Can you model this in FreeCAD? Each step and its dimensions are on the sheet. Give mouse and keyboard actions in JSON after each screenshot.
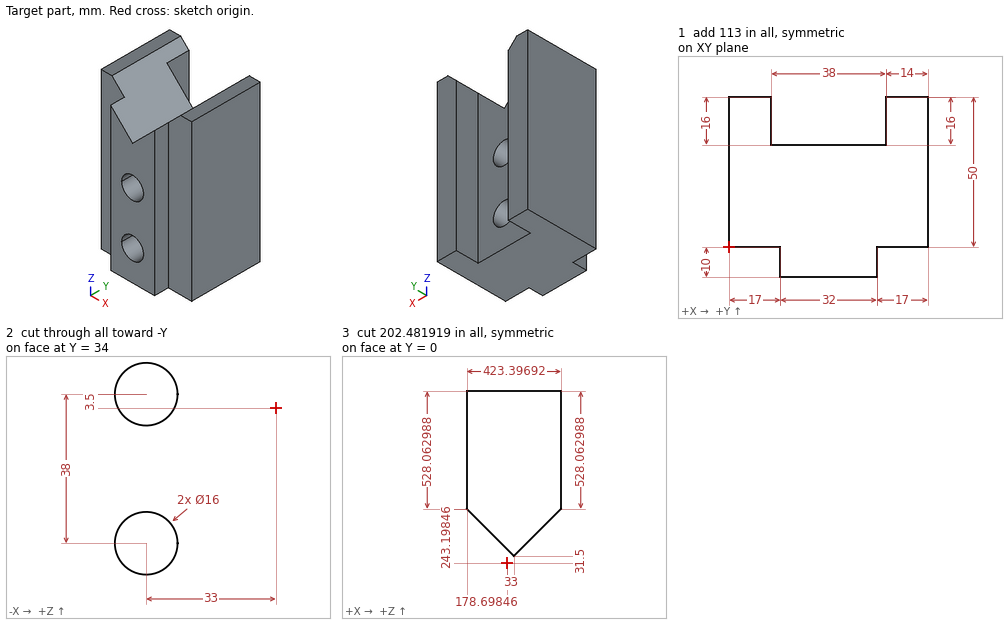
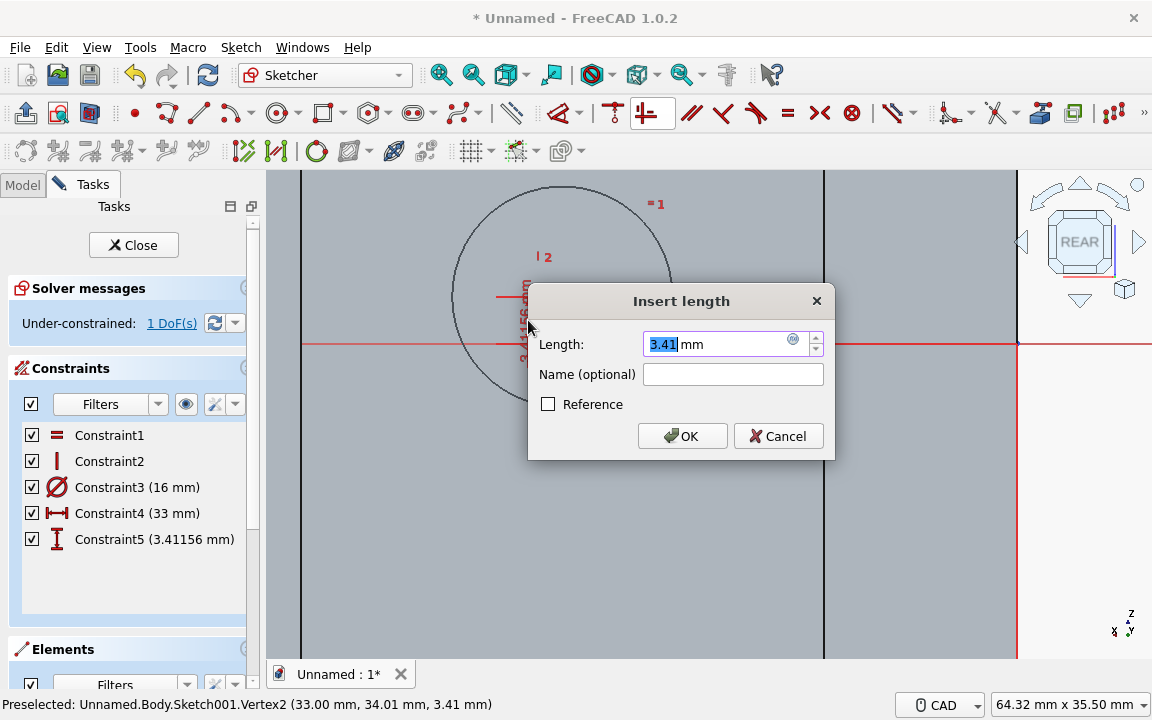
{"action": "type", "text": "3.5"}
{"action": "key", "text": "Return"}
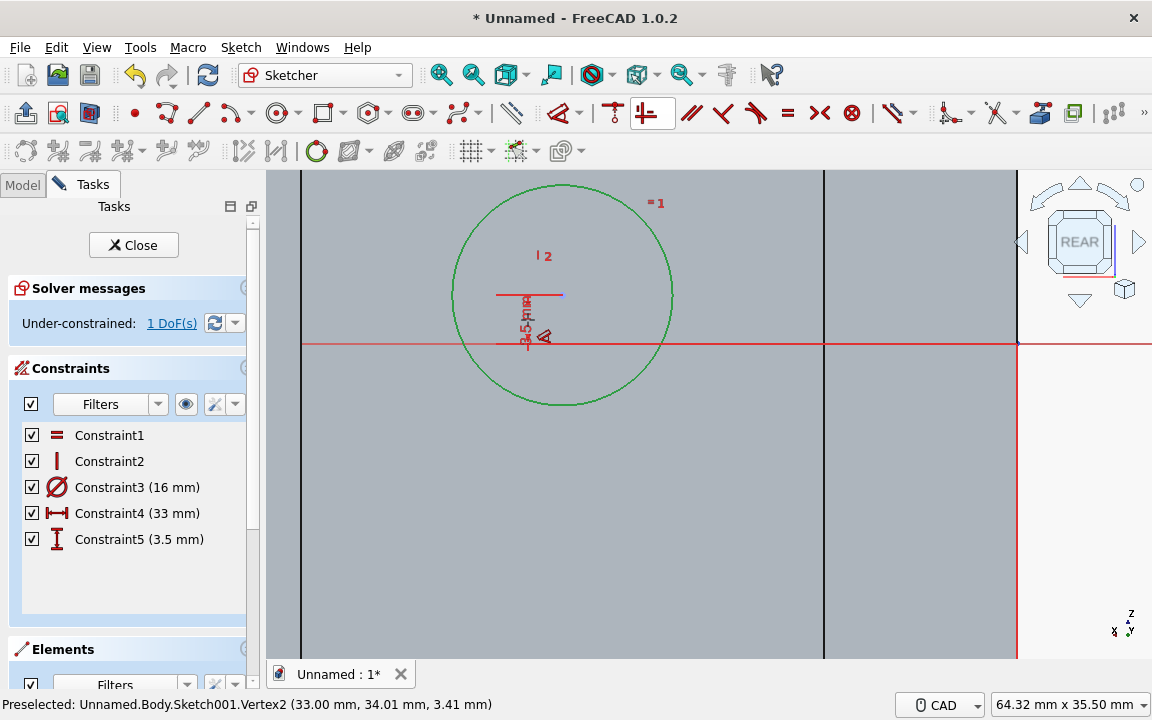
{"action": "scroll", "coordinate": [564, 298], "scroll_direction": "down", "scroll_amount": 4}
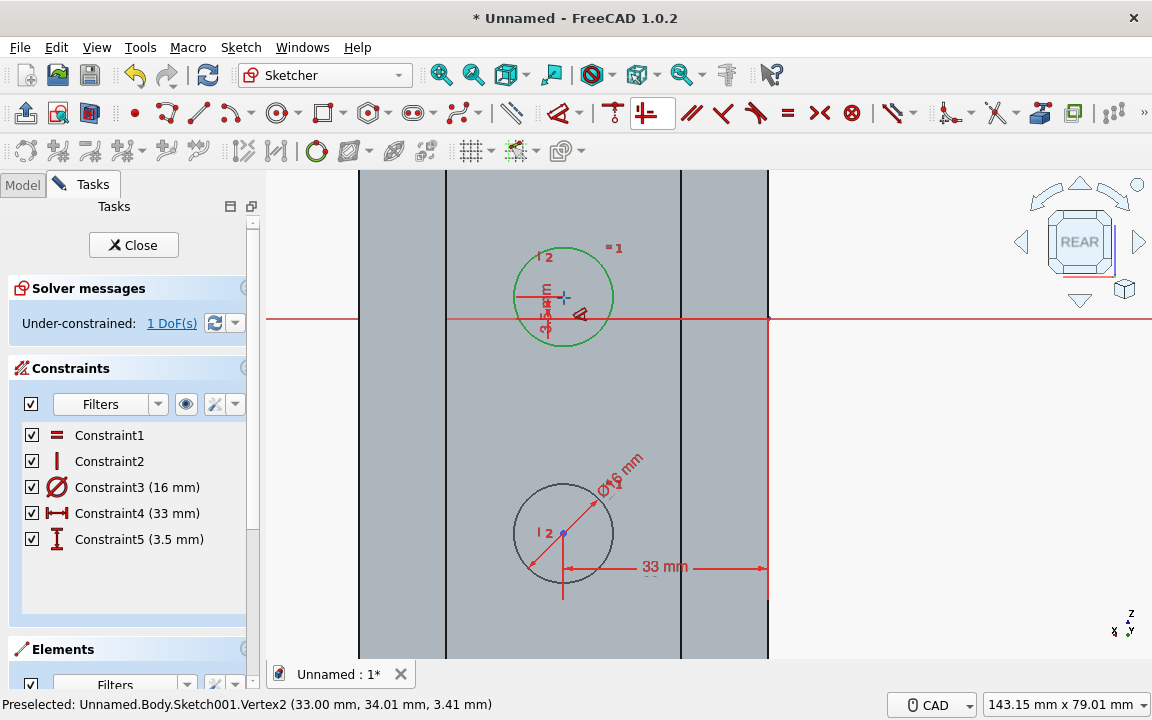
{"action": "left_click", "coordinate": [563, 534]}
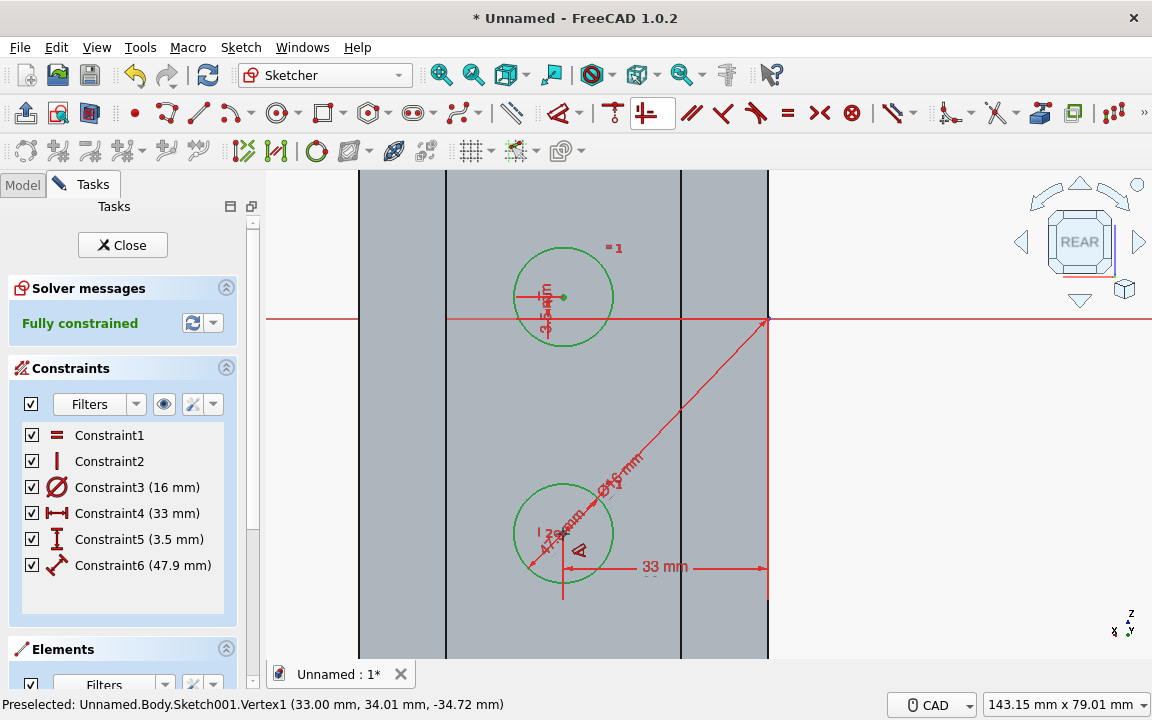
{"action": "left_click", "coordinate": [563, 297]}
{"action": "left_click", "coordinate": [529, 415]}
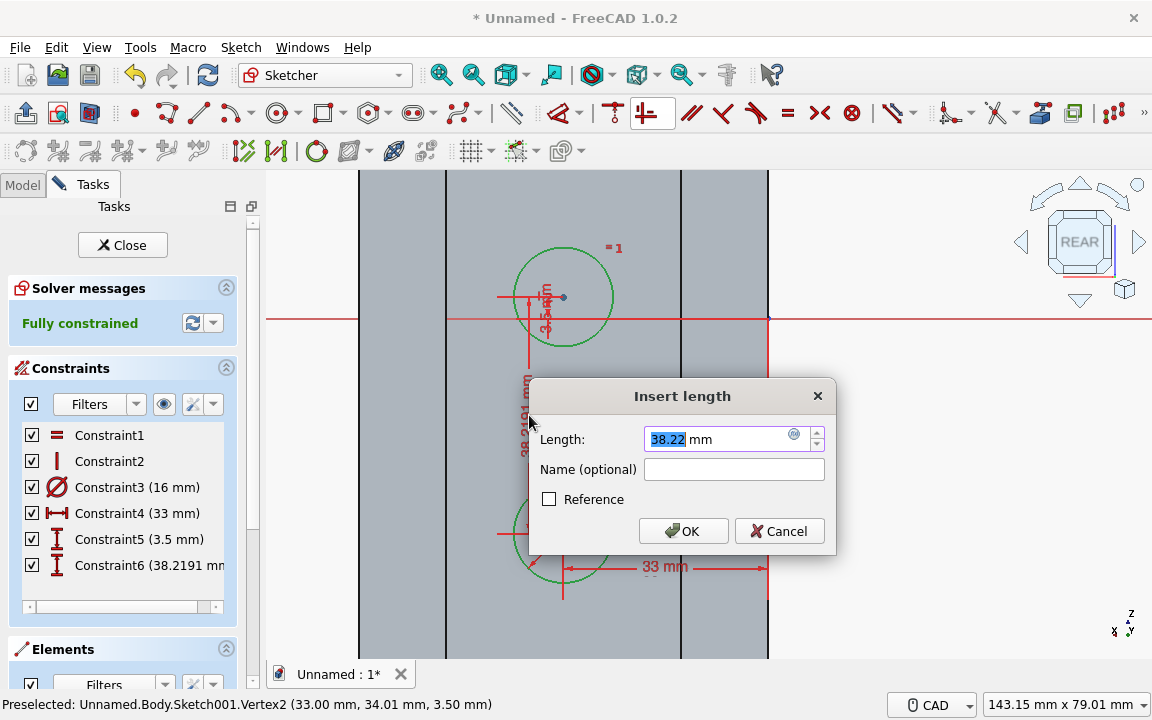
{"action": "type", "text": "38"}
{"action": "key", "text": "Return"}
{"action": "key", "text": "Escape"}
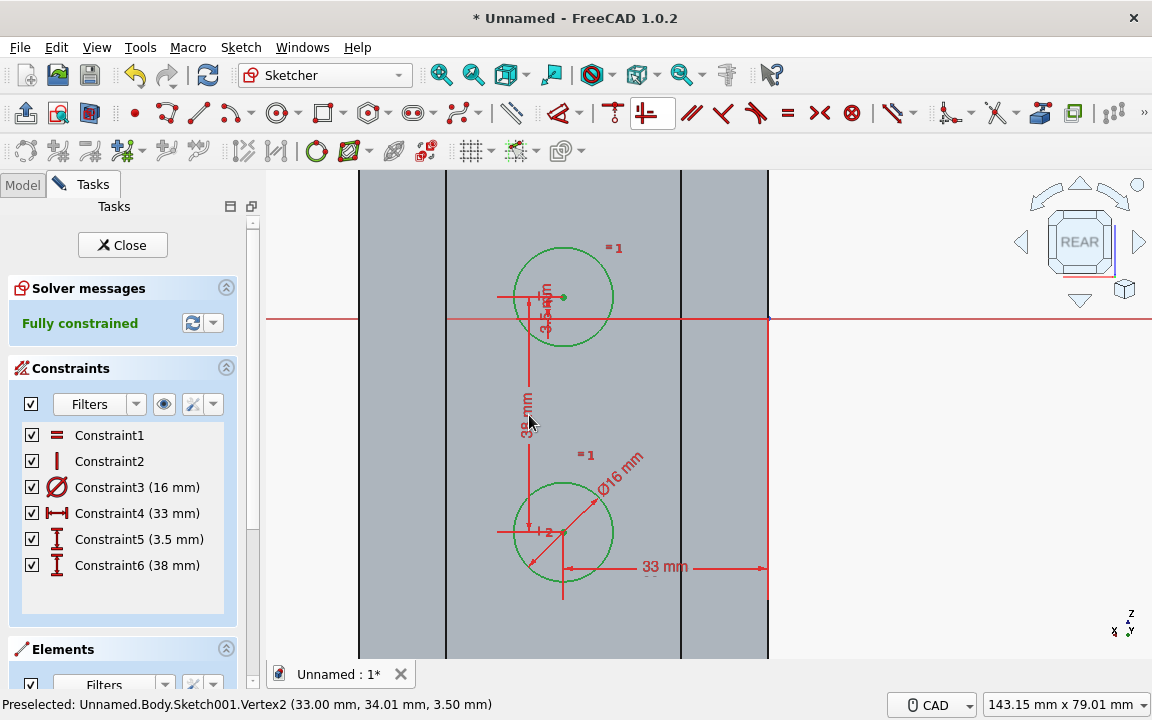
{"action": "left_click", "coordinate": [123, 245]}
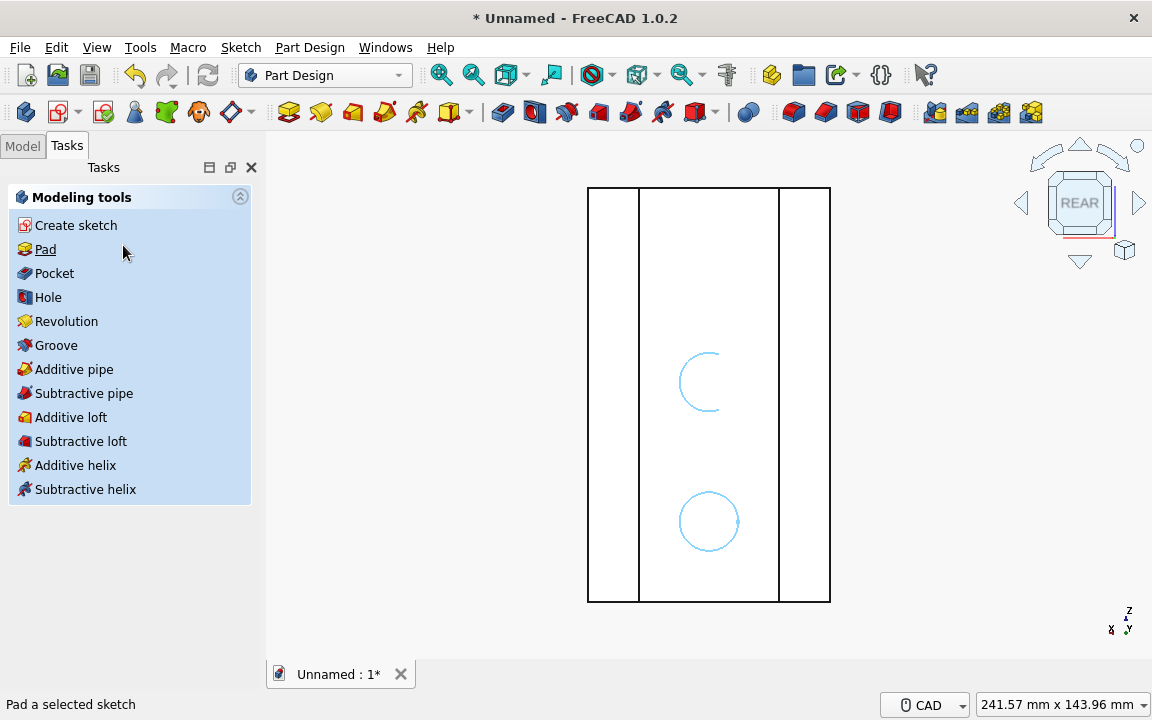
{"action": "left_click", "coordinate": [504, 112]}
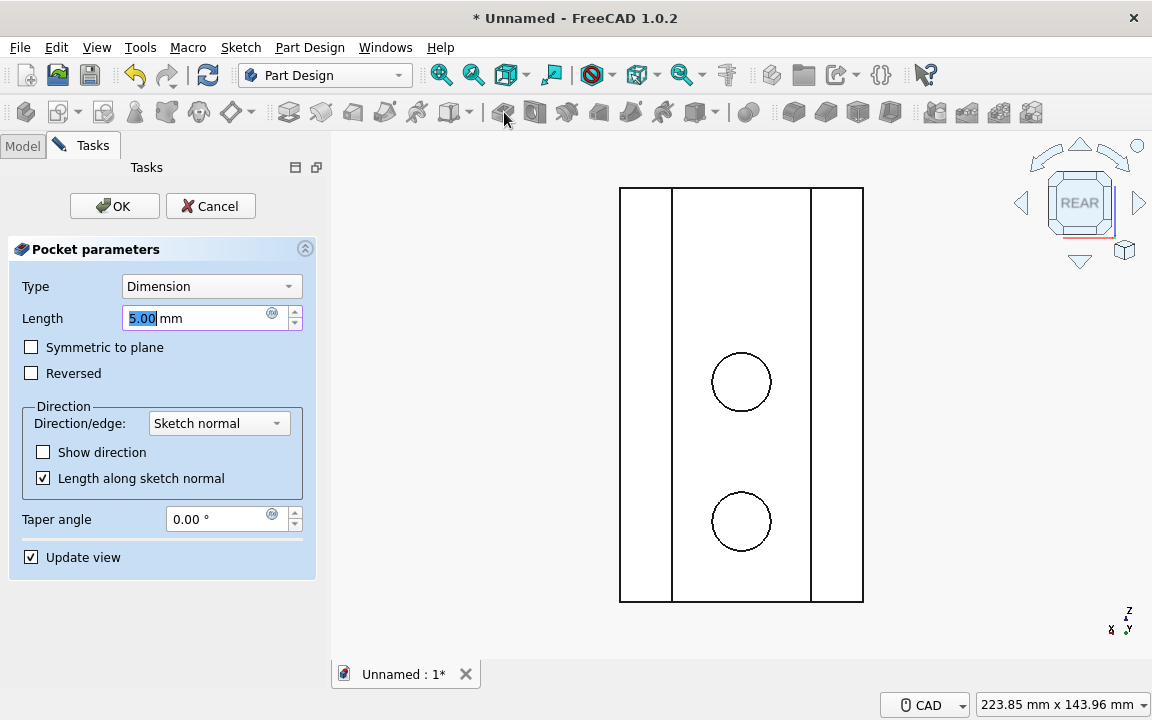
{"action": "left_click", "coordinate": [212, 286]}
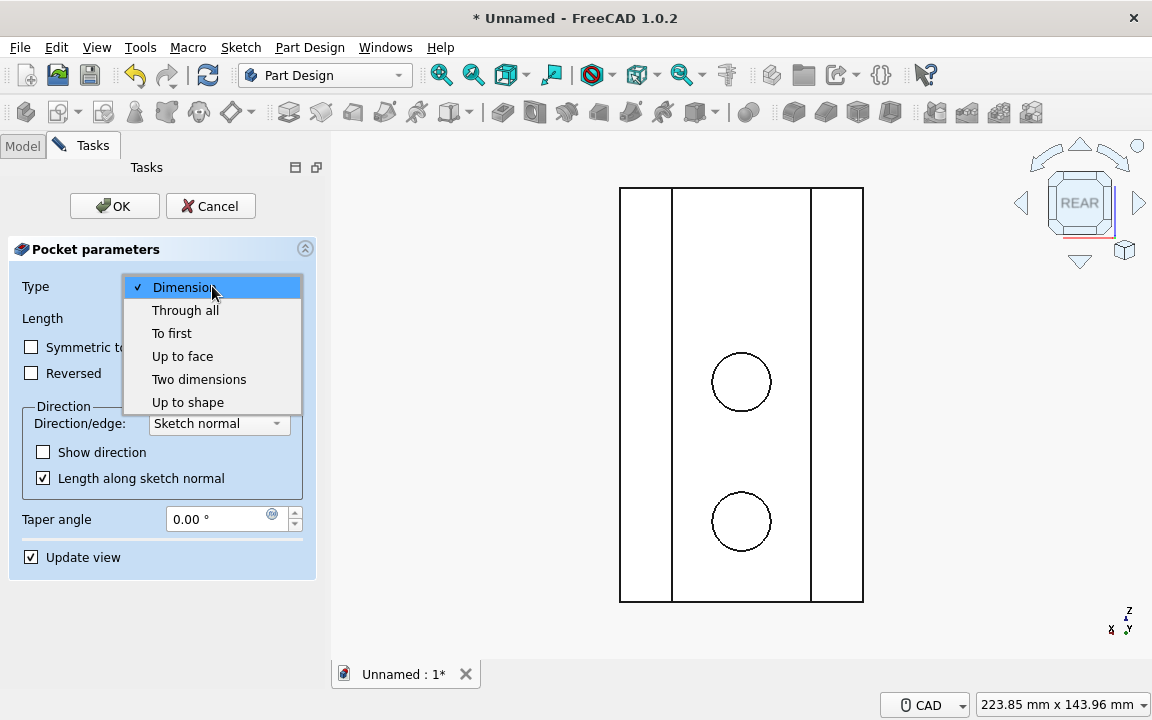
{"action": "left_click", "coordinate": [212, 310]}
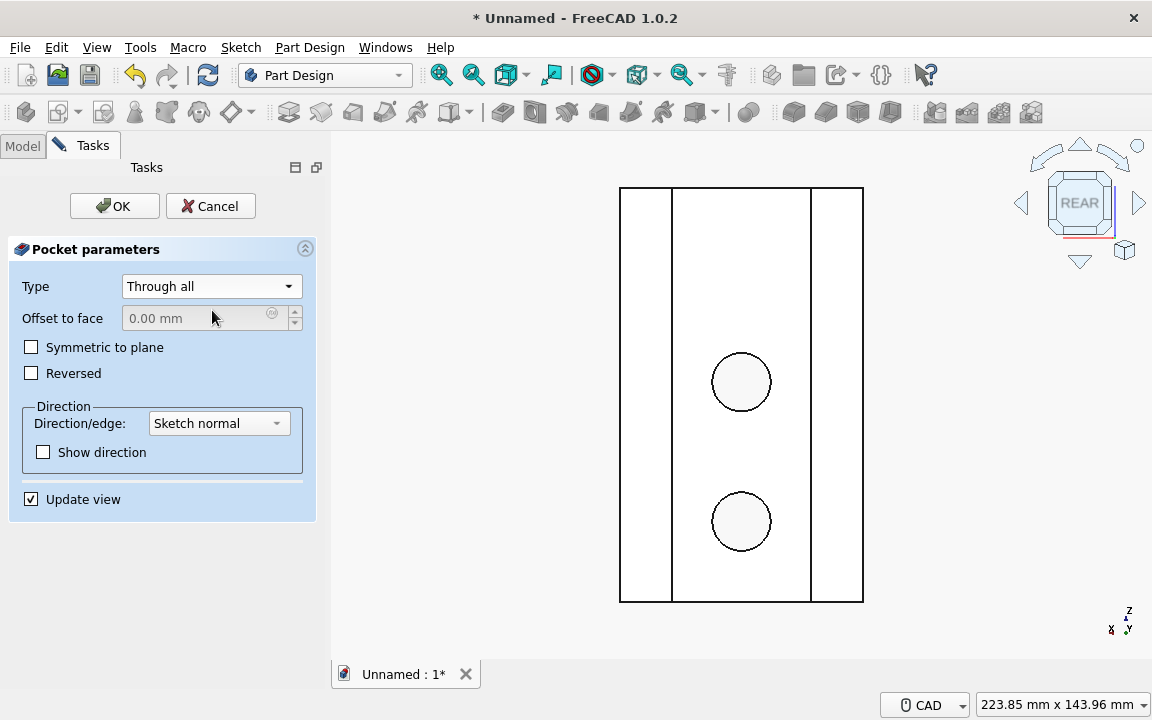
{"action": "left_click", "coordinate": [115, 206]}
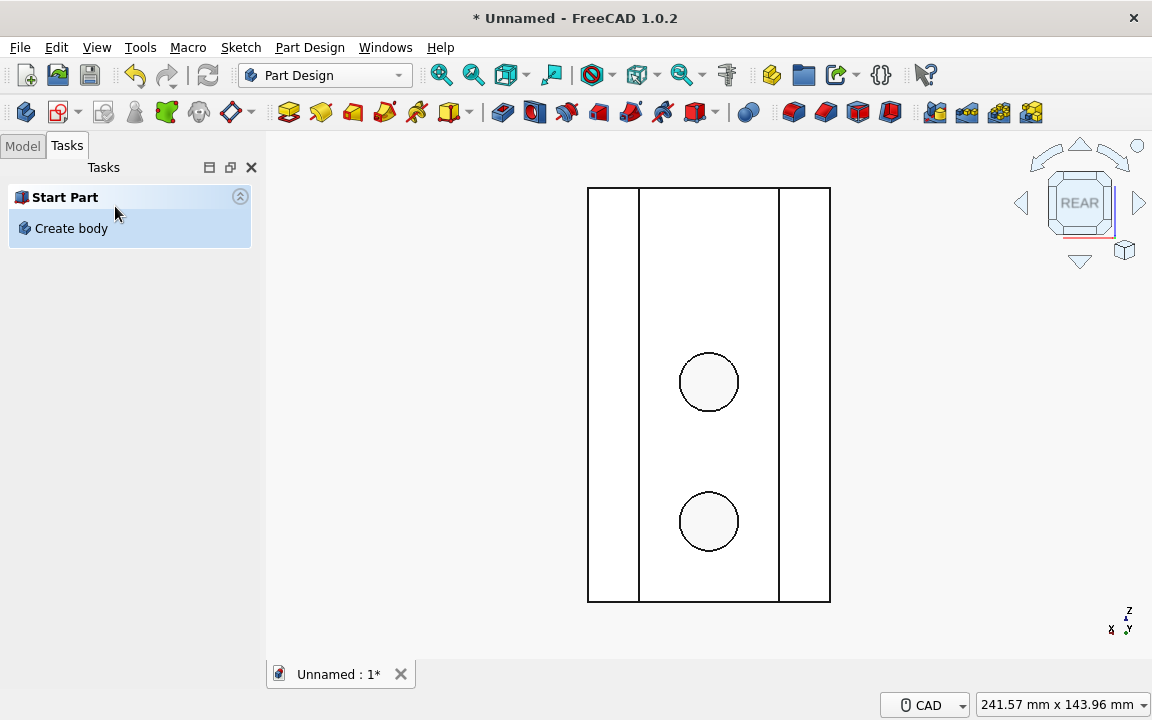
{"action": "key", "text": "0"}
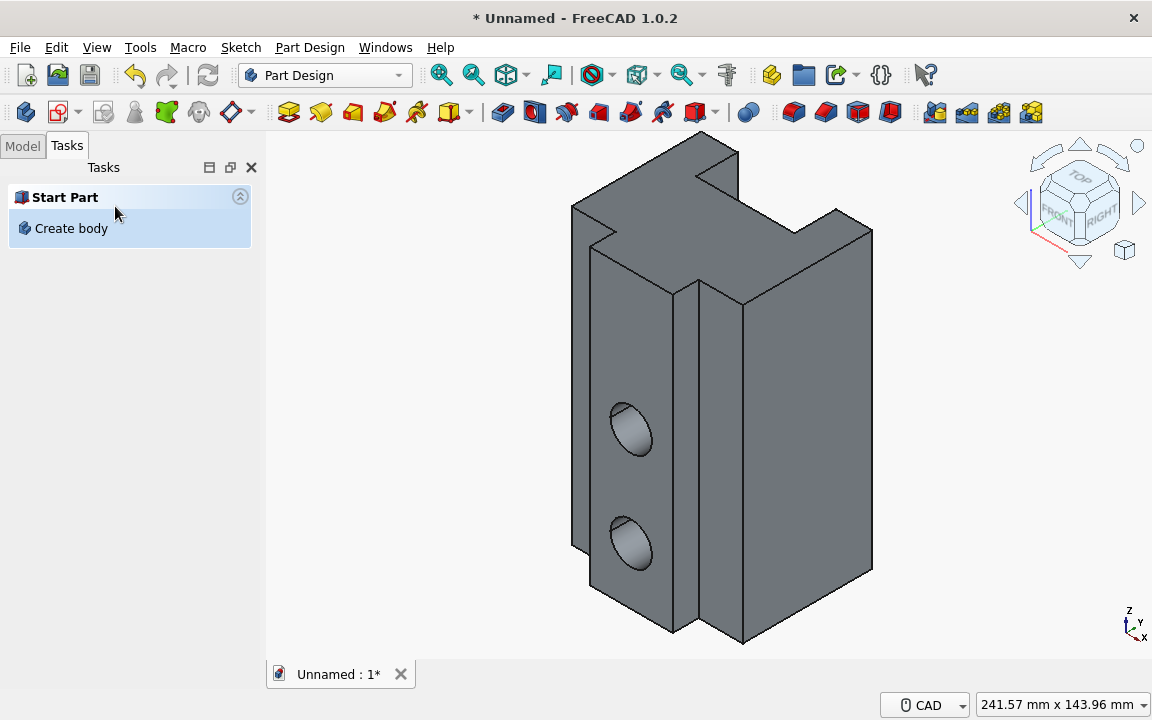
{"action": "left_click", "coordinate": [442, 76]}